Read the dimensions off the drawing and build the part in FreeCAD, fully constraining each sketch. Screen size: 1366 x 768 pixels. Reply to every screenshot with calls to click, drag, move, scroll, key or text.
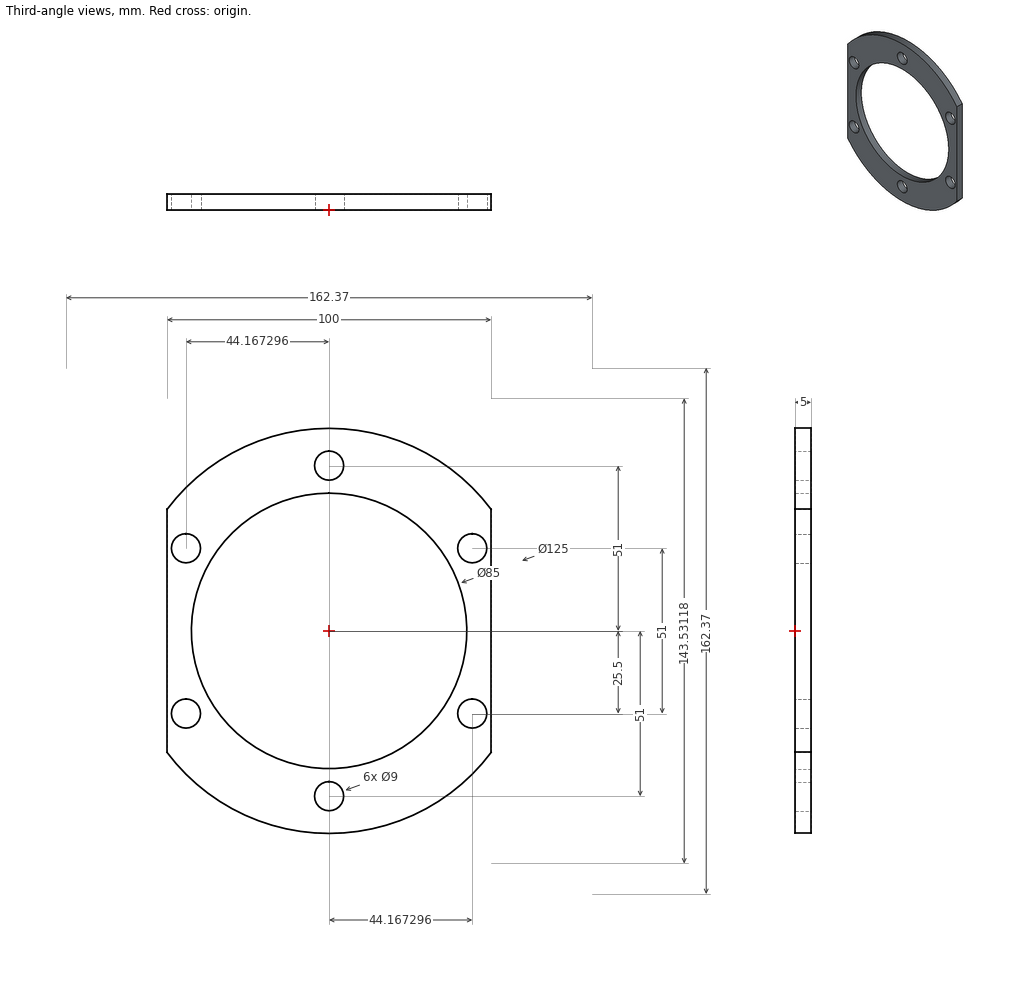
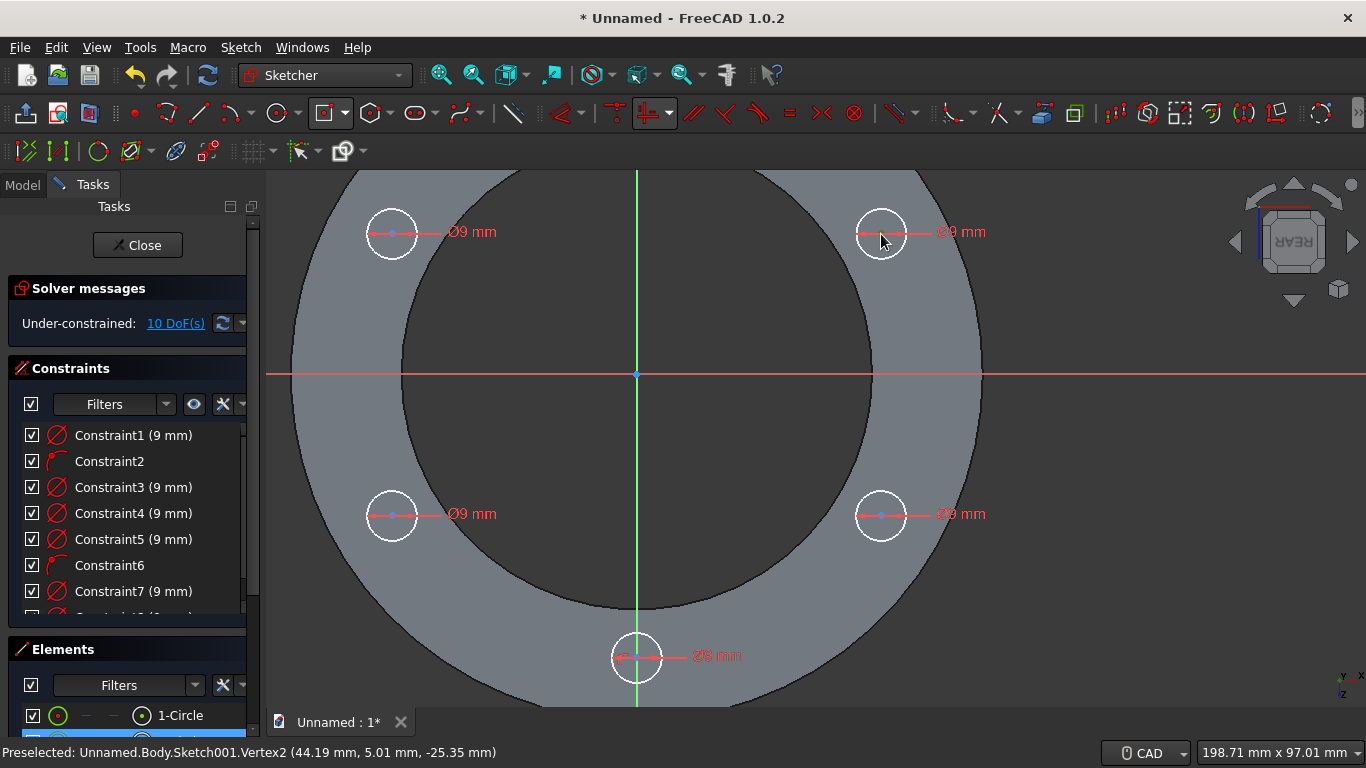
click(881, 516)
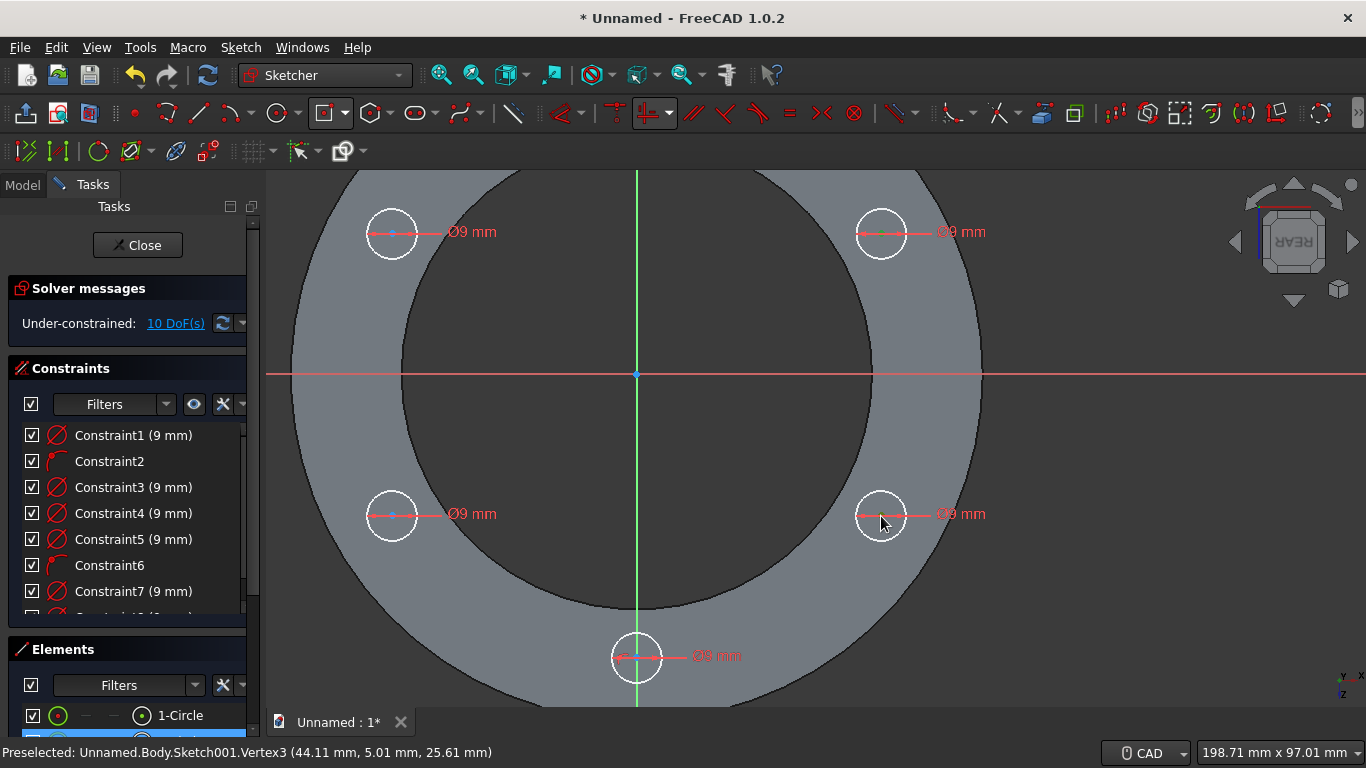
key(v)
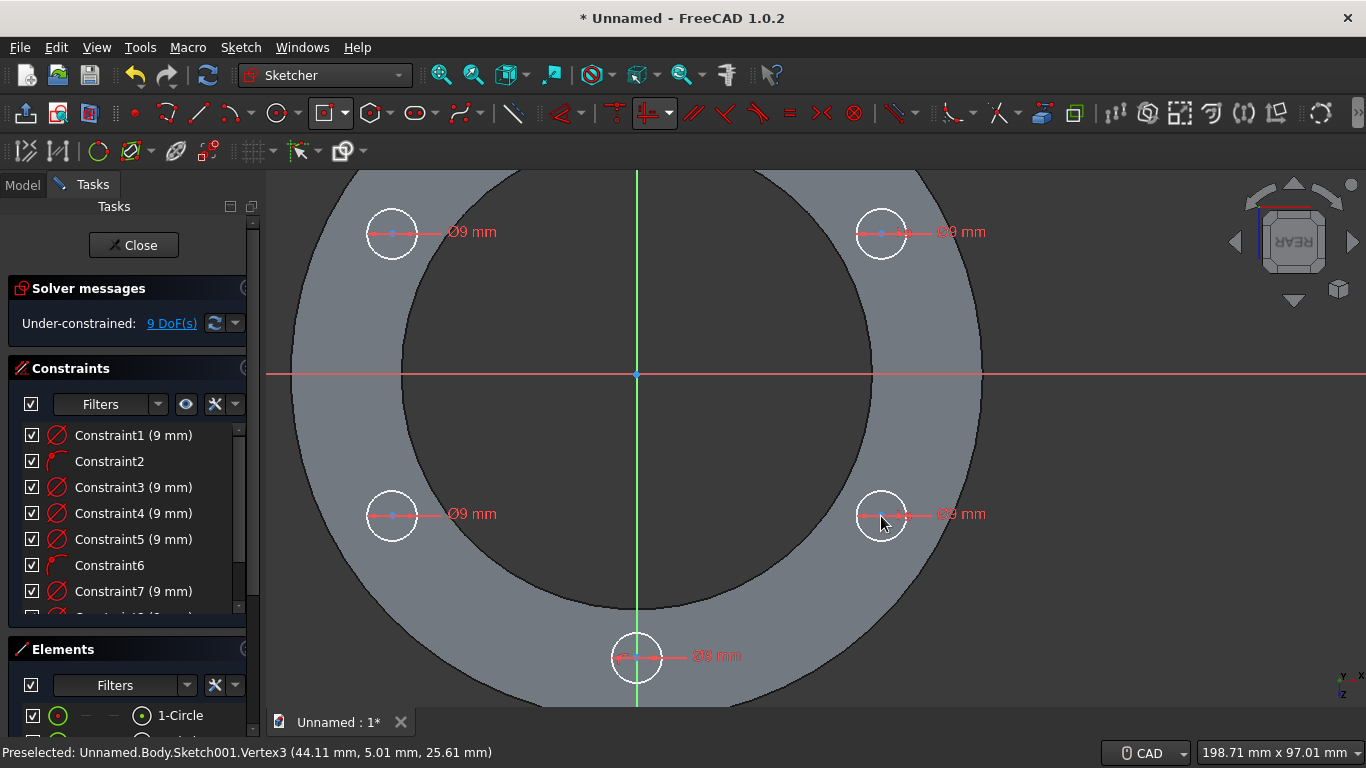
click(881, 516)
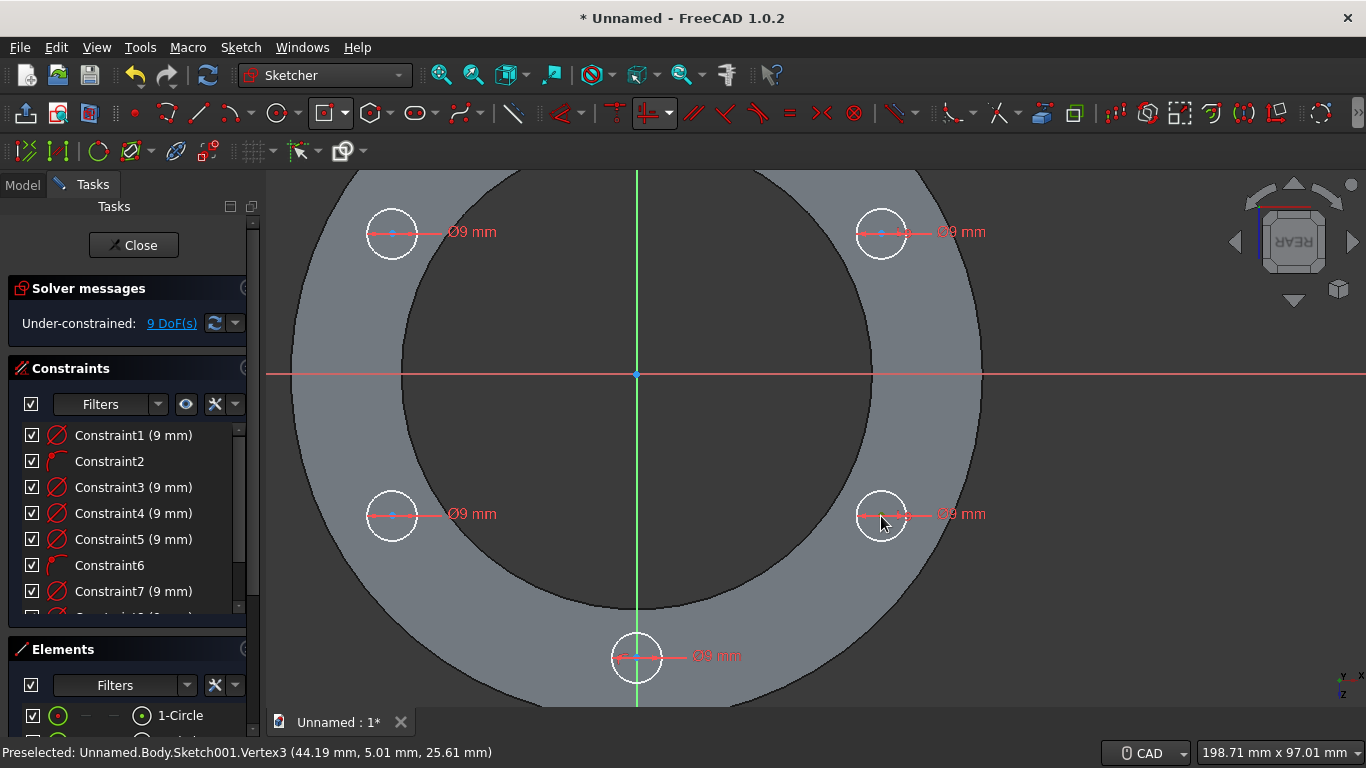
click(392, 516)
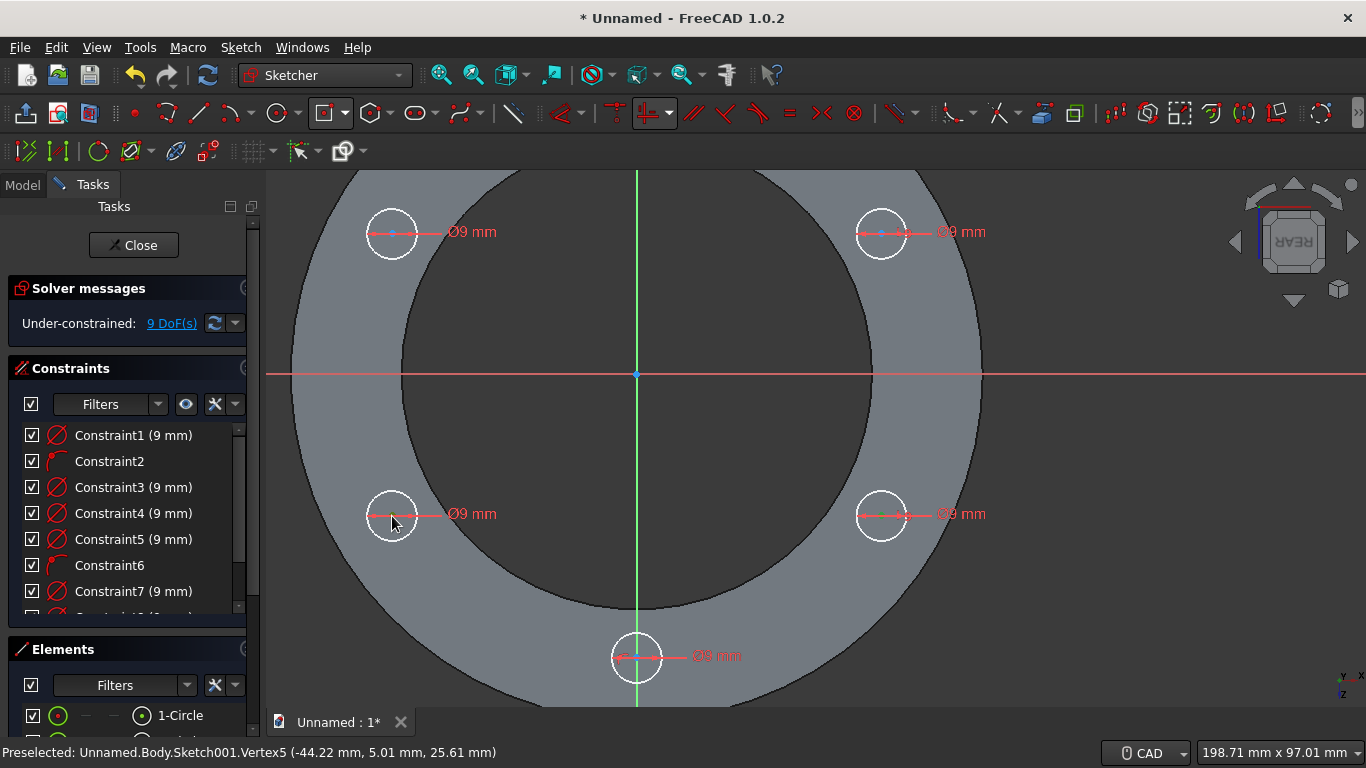
click(672, 114)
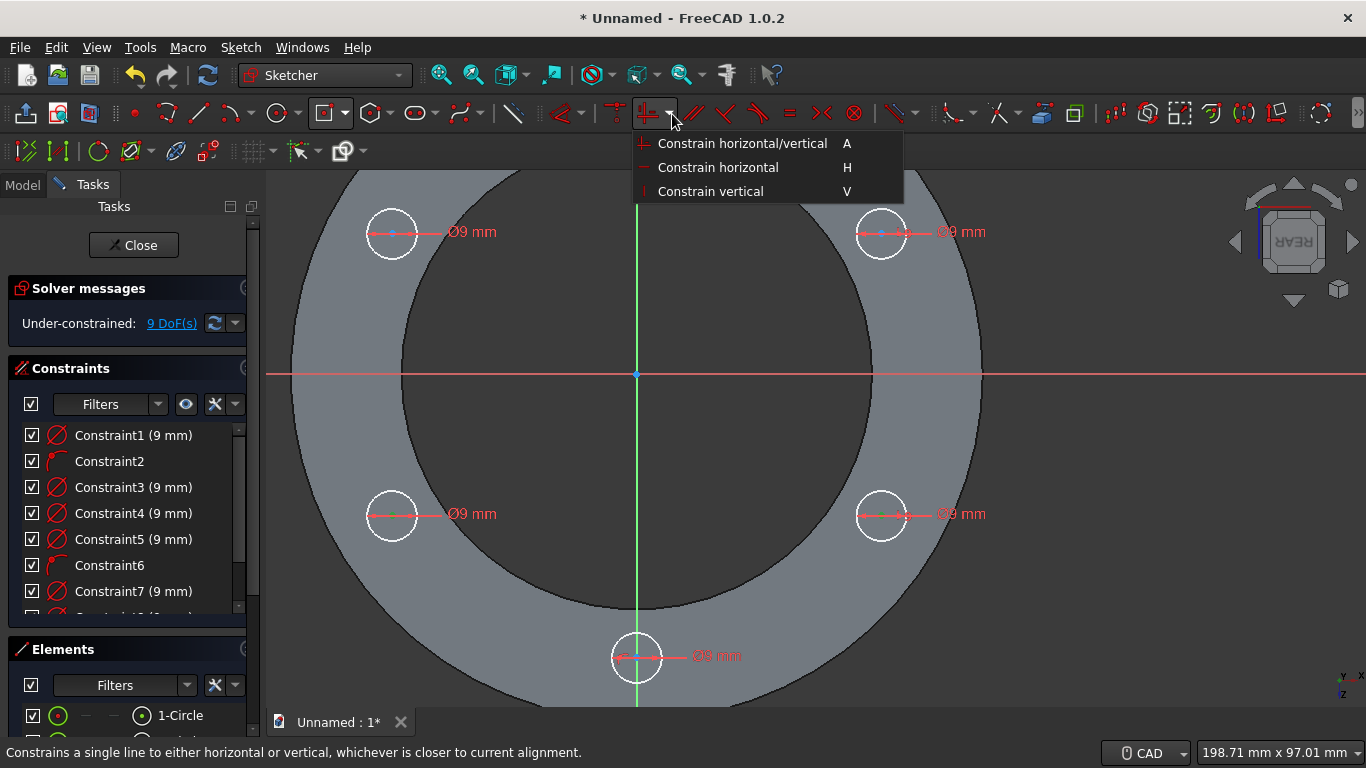
click(768, 167)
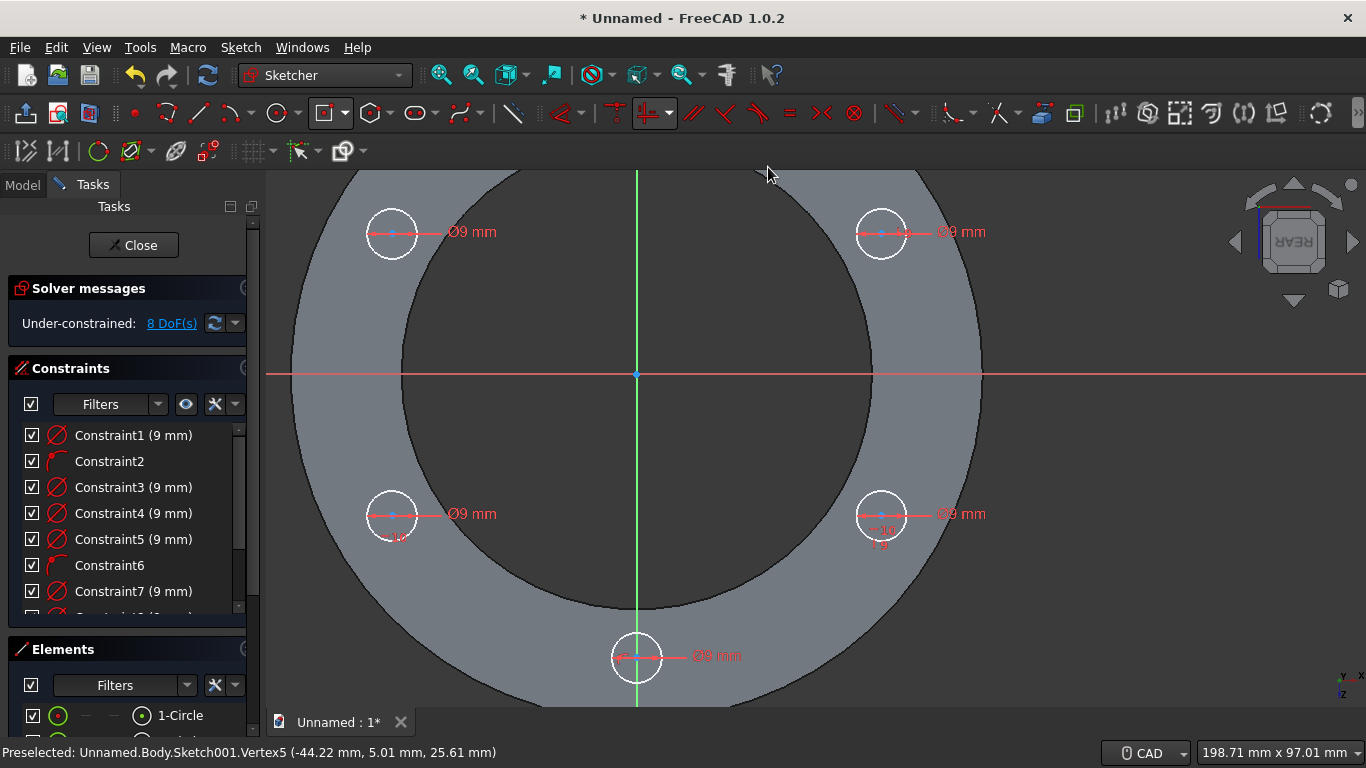
click(392, 516)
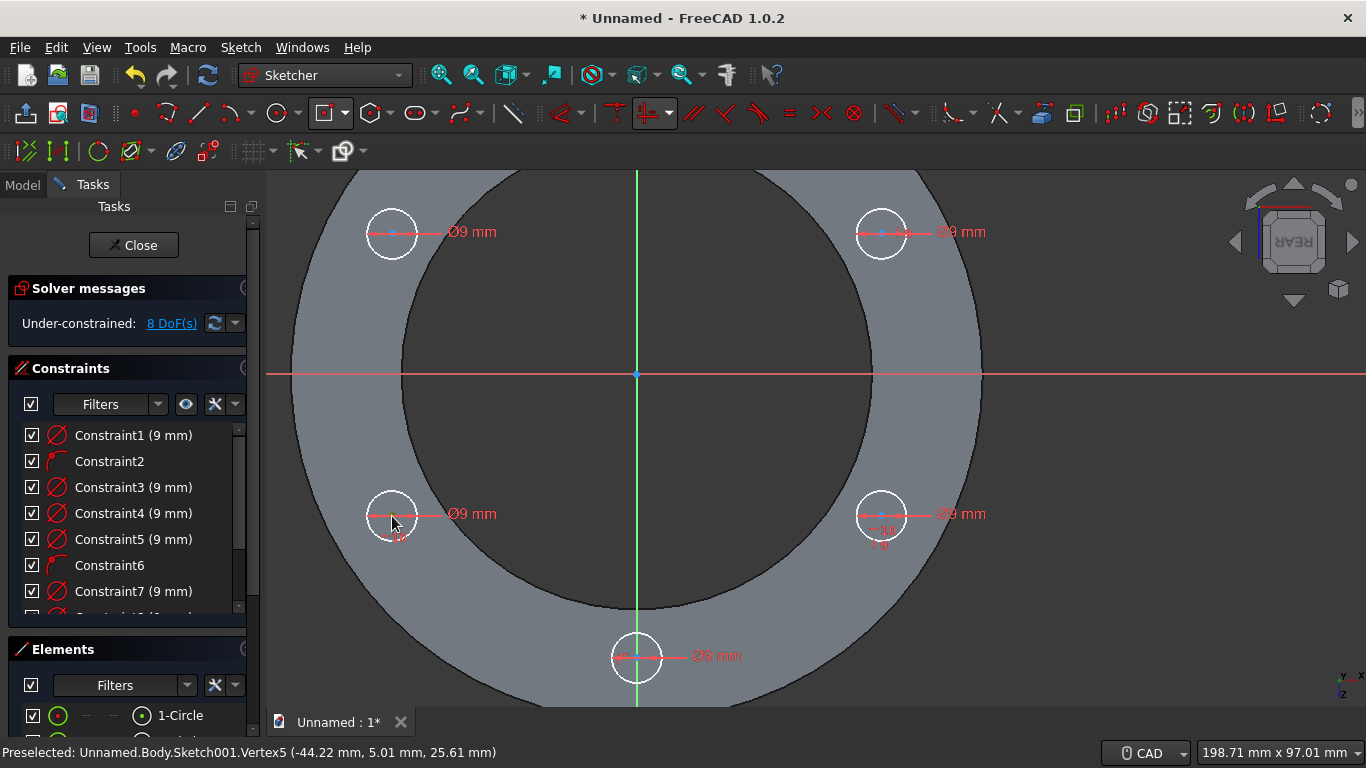
click(392, 234)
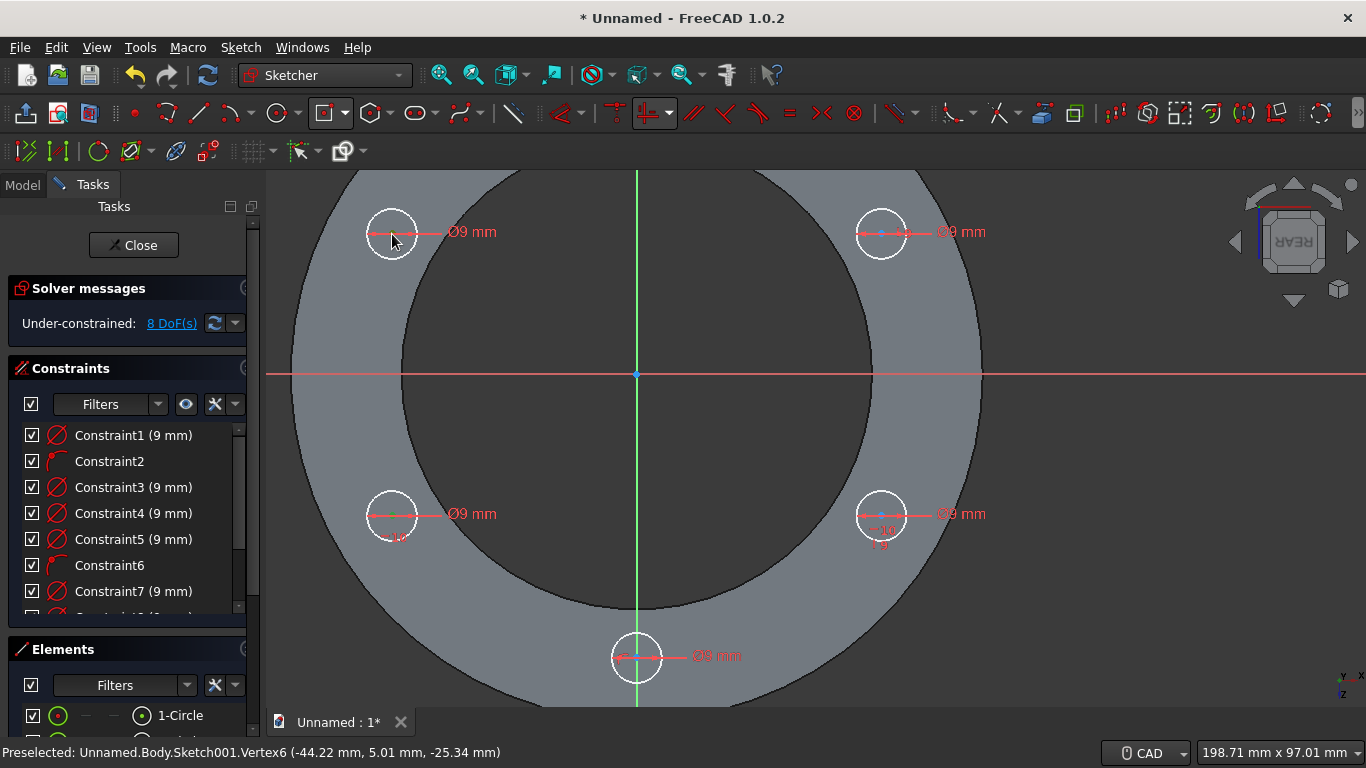
click(672, 114)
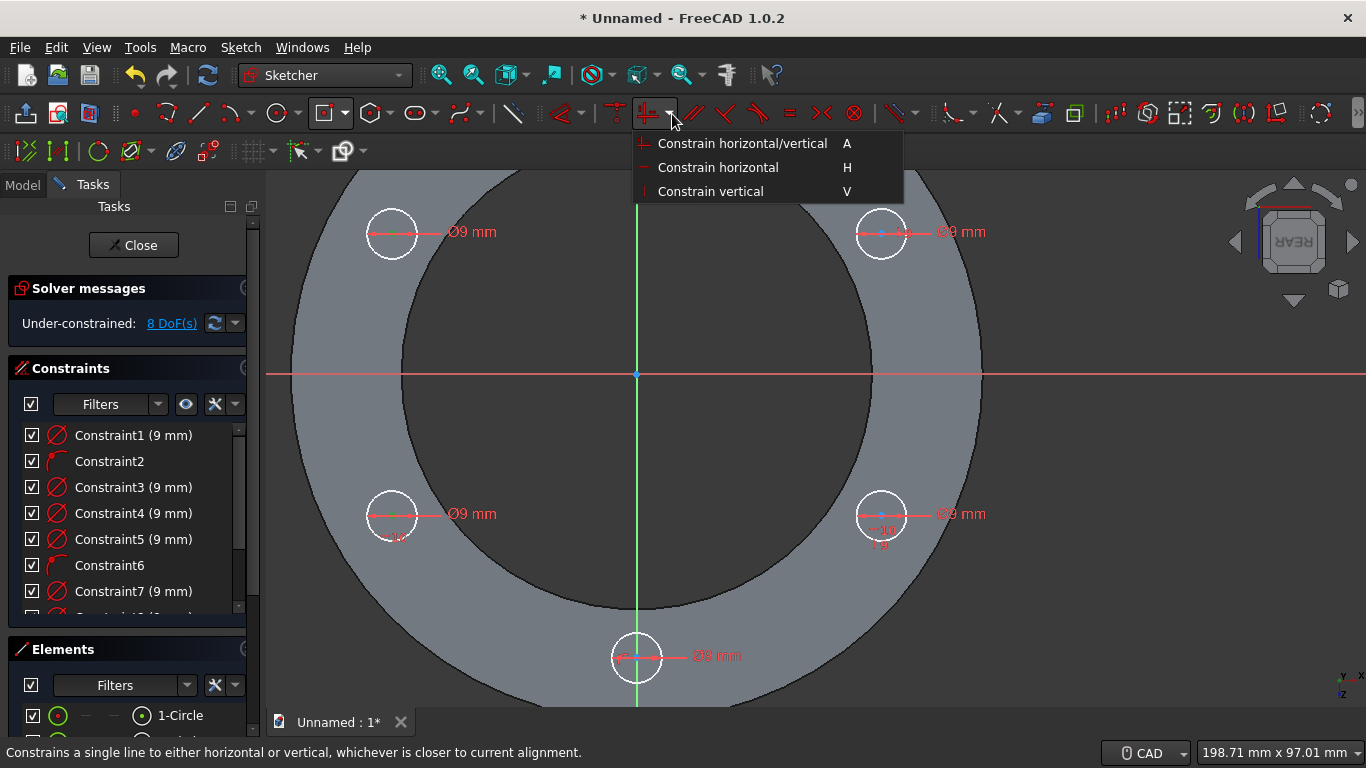
click(768, 191)